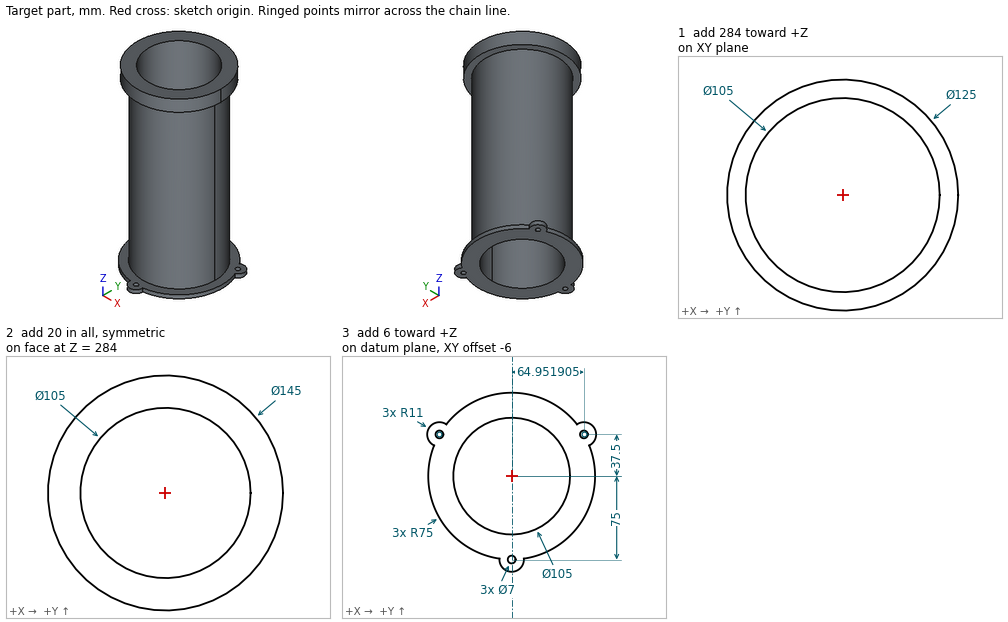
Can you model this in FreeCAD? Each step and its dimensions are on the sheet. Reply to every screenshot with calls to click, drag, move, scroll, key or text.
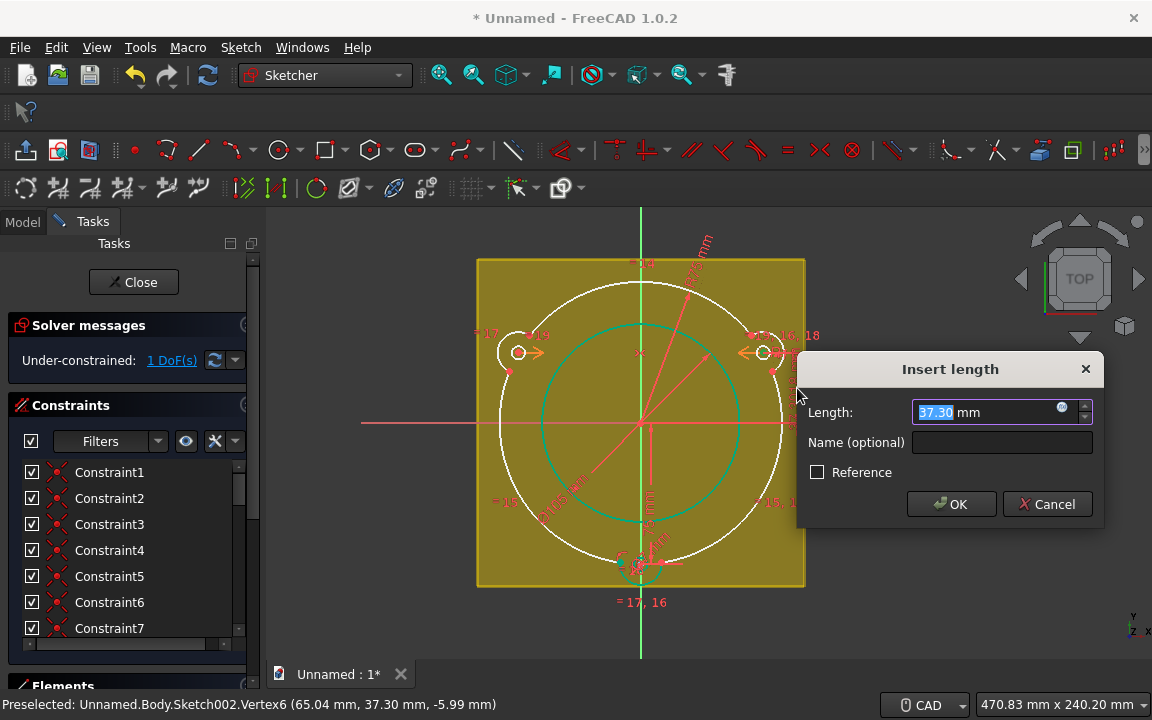
text(37.5)
key(Return)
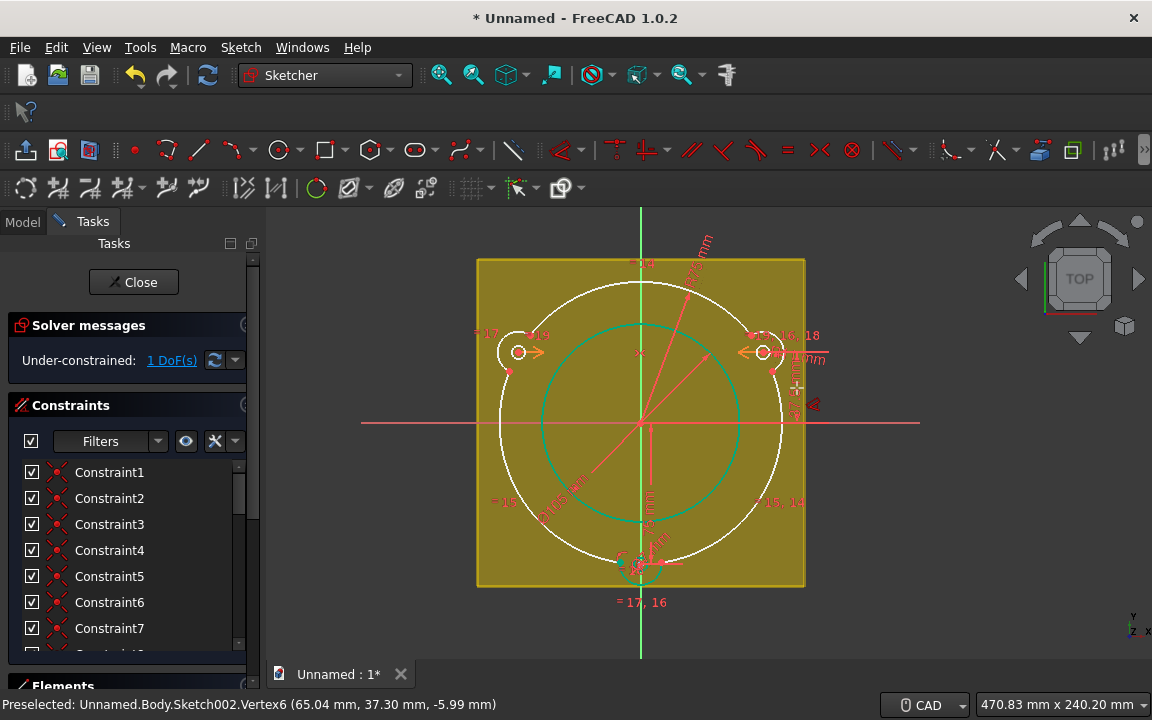
click(763, 352)
click(702, 318)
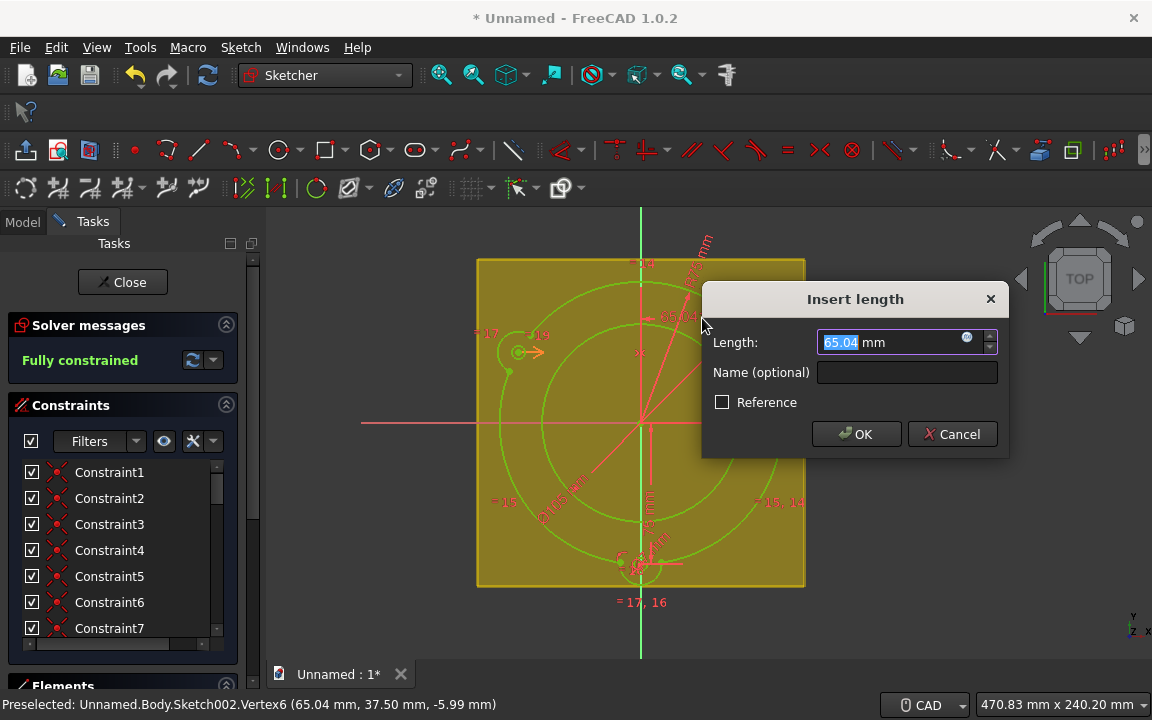
text(64.951905)
key(Return)
key(Escape)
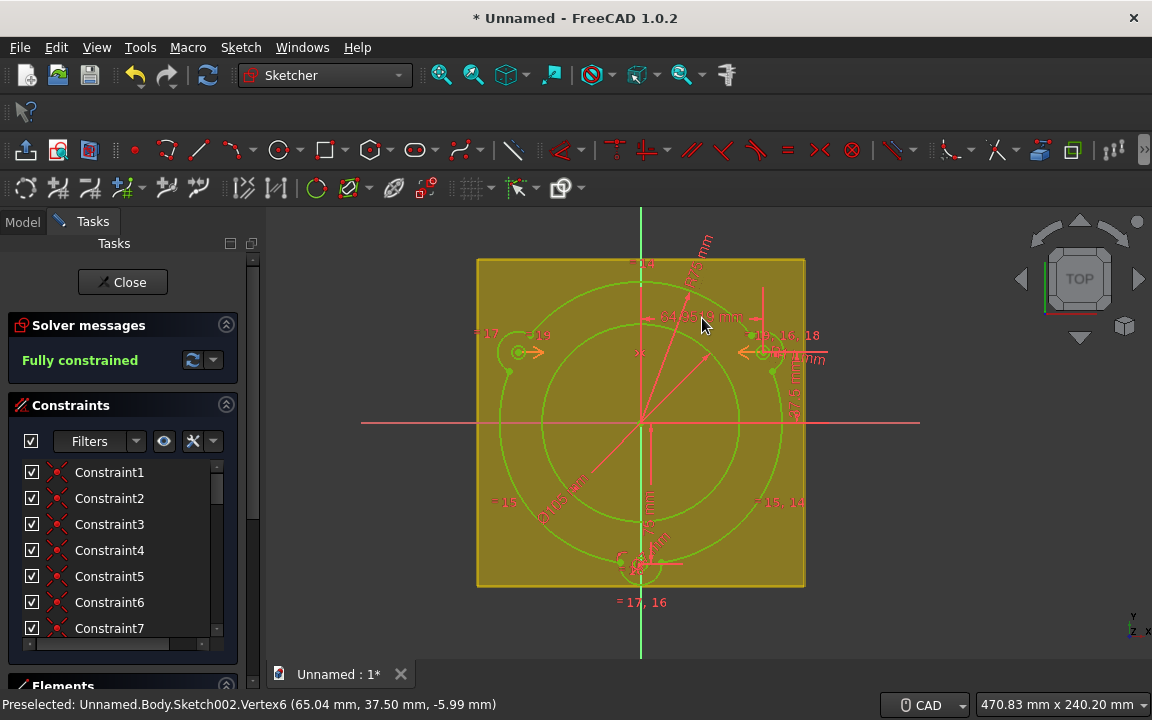
click(123, 282)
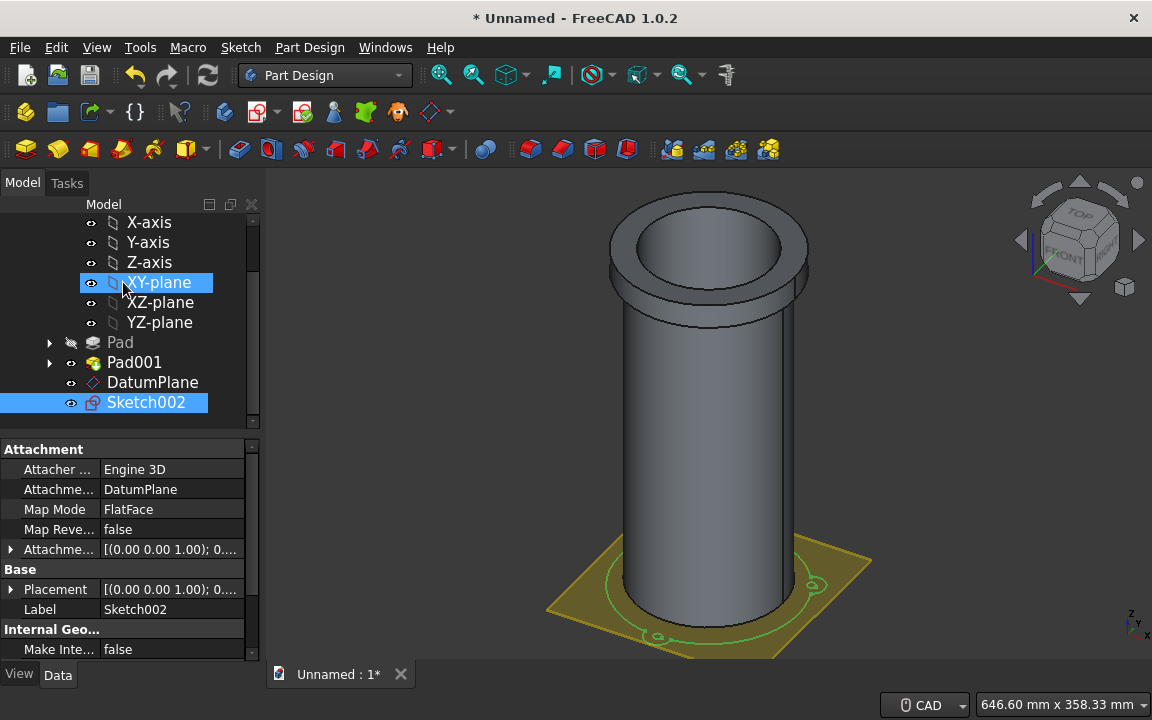
click(26, 150)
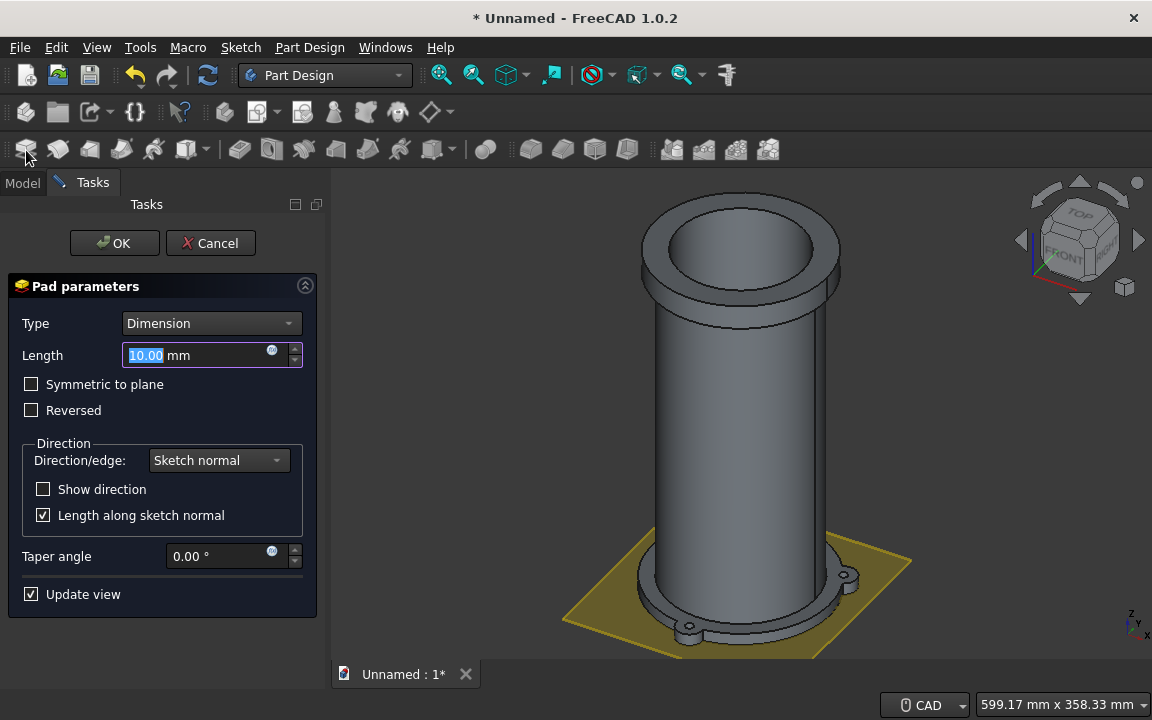
text(6)
key(Tab)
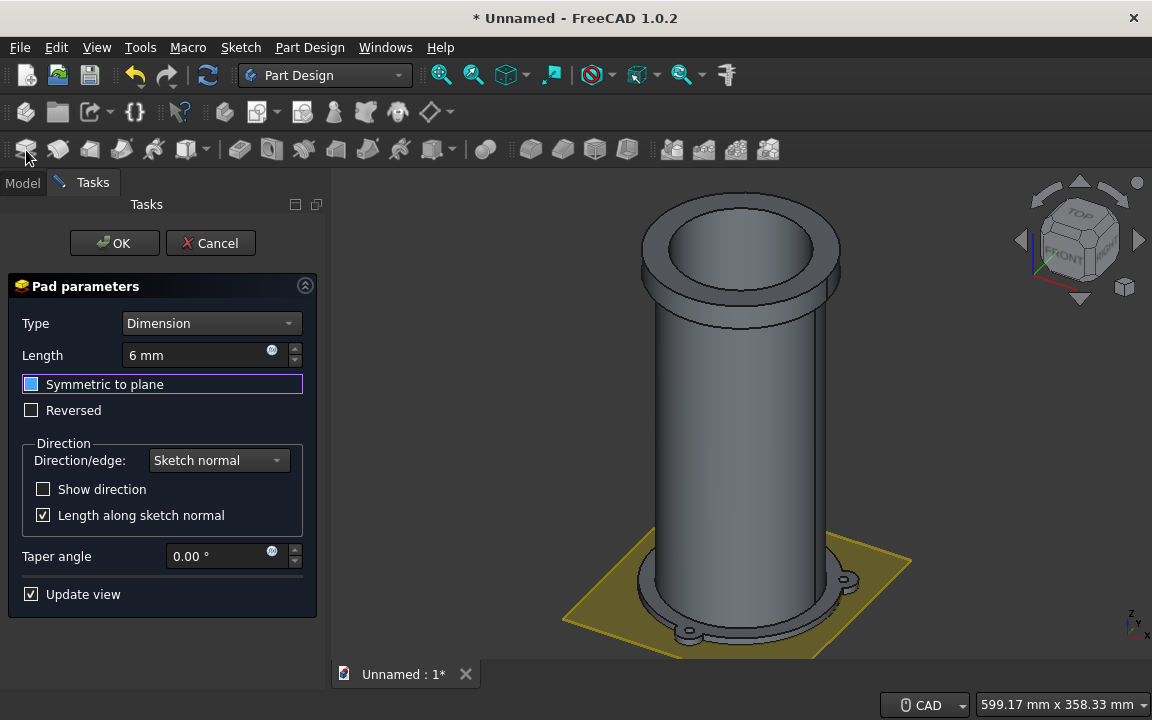
click(115, 243)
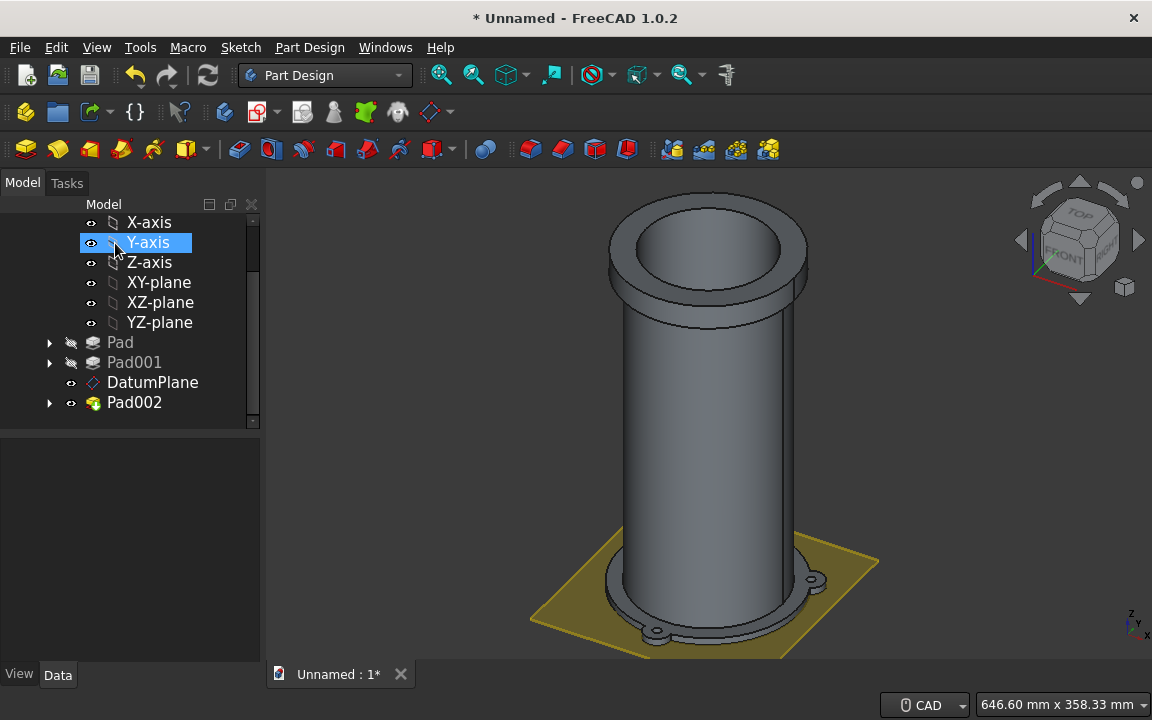
click(116, 383)
key(space)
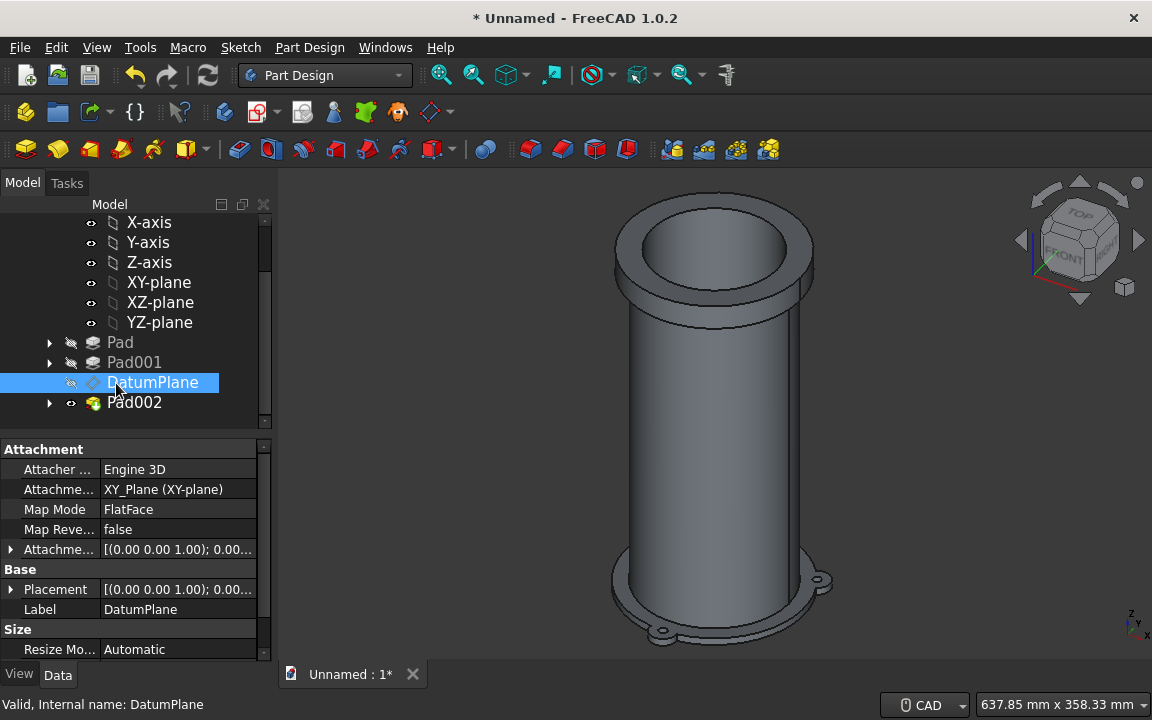
key(0)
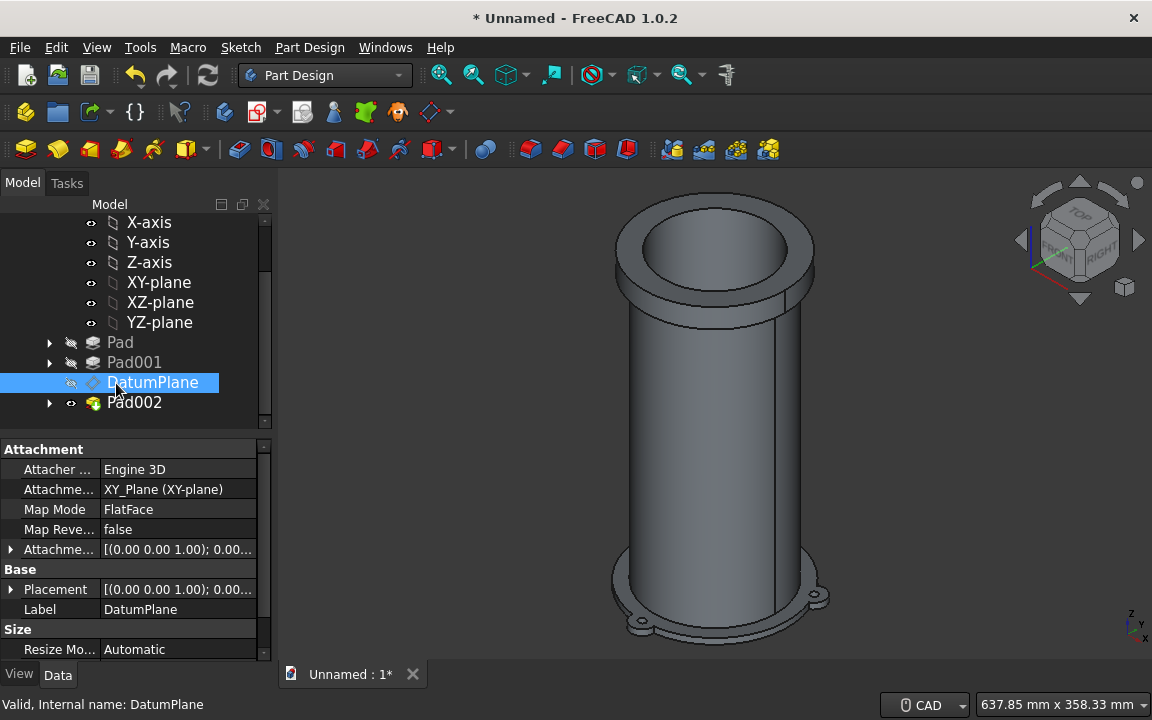
click(442, 76)